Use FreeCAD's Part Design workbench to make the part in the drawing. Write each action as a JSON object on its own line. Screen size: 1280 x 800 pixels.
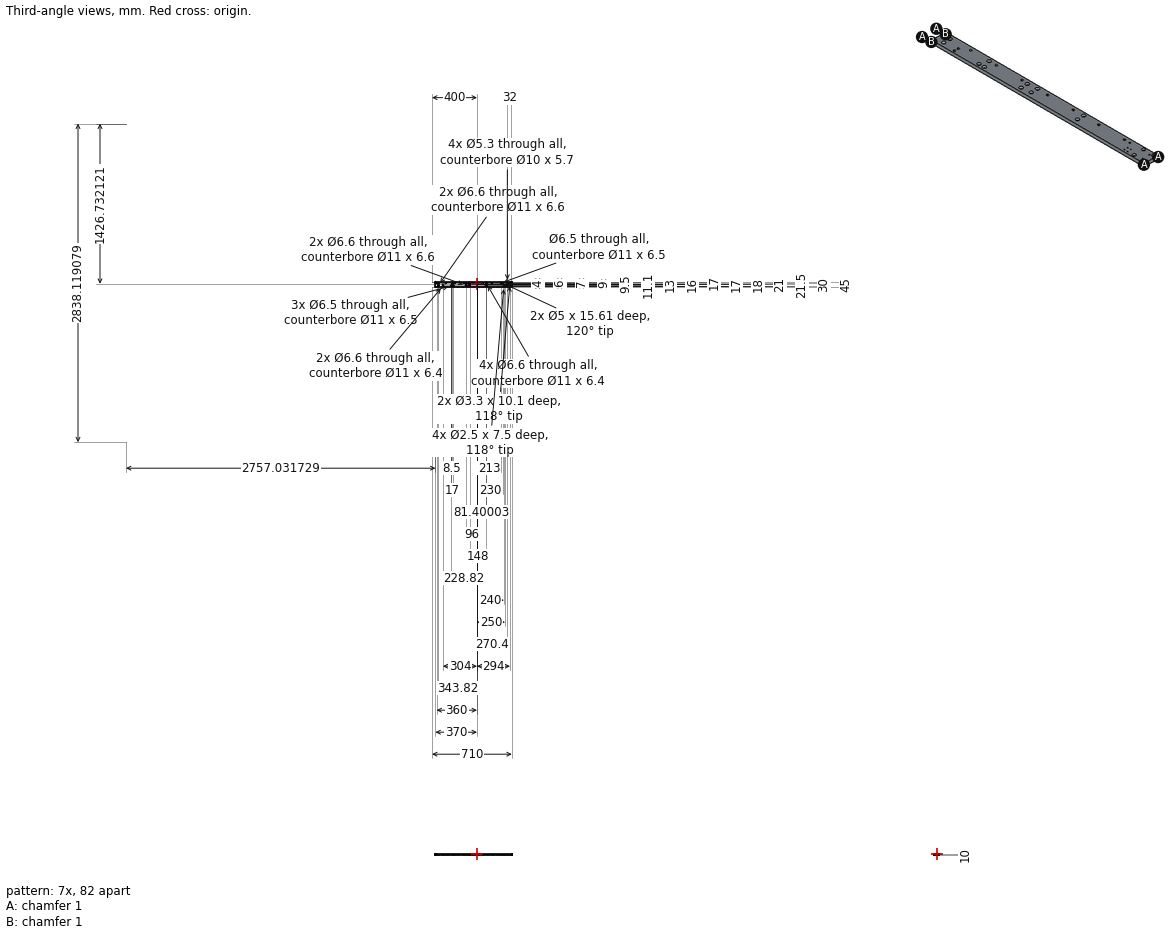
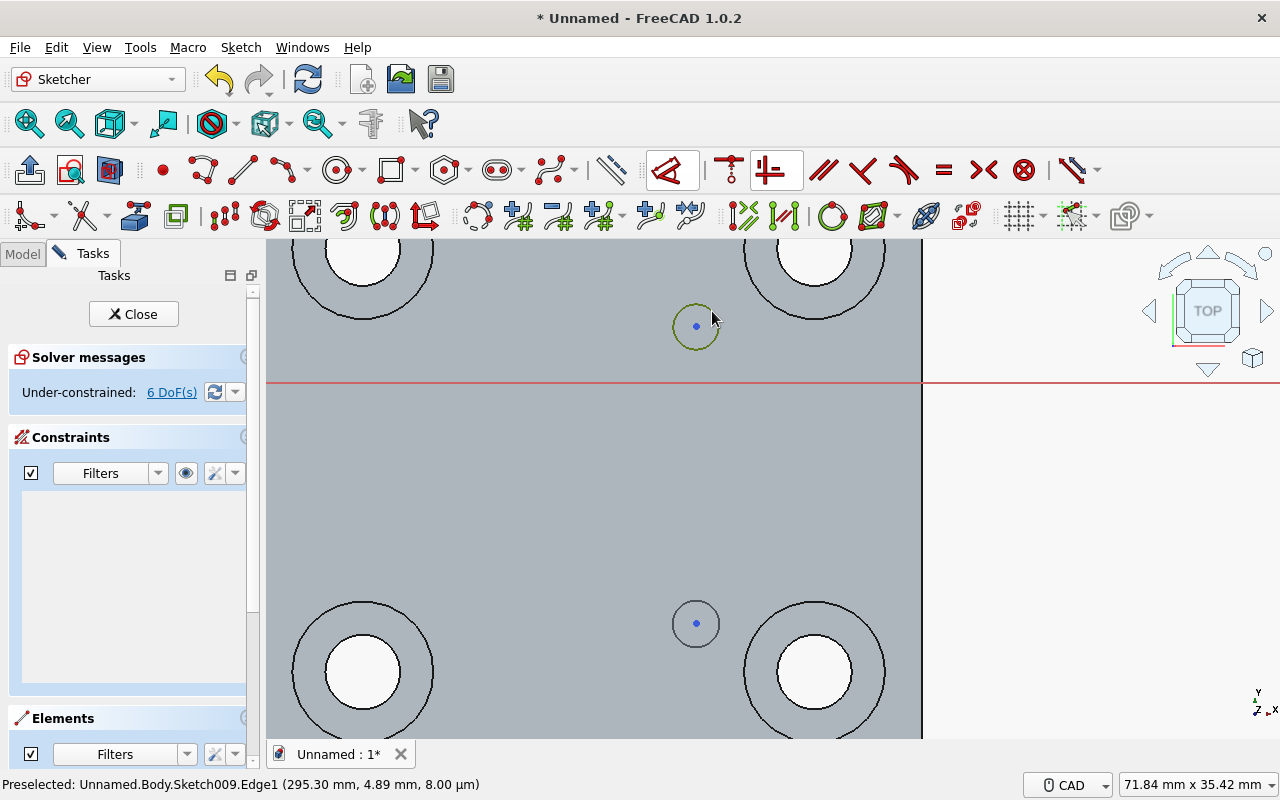
{"action": "left_click", "coordinate": [712, 607]}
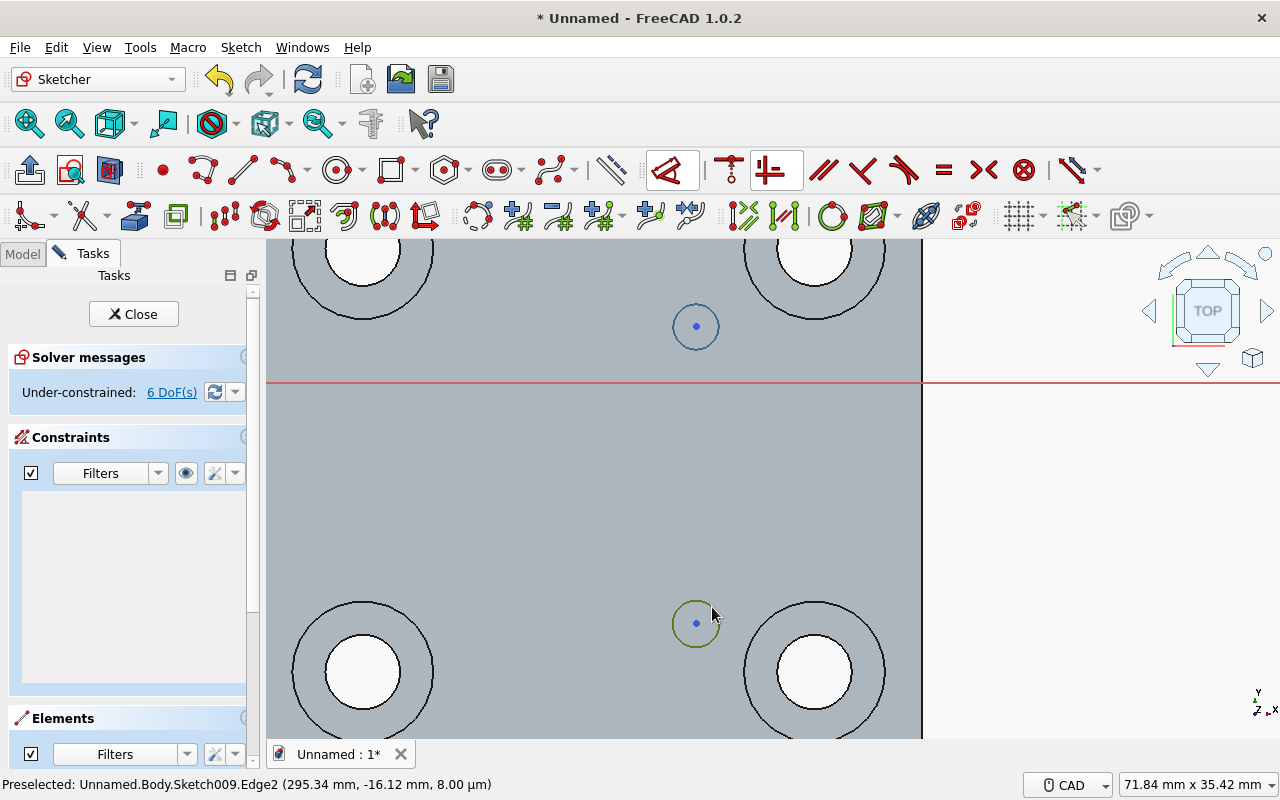
{"action": "left_click", "coordinate": [944, 170]}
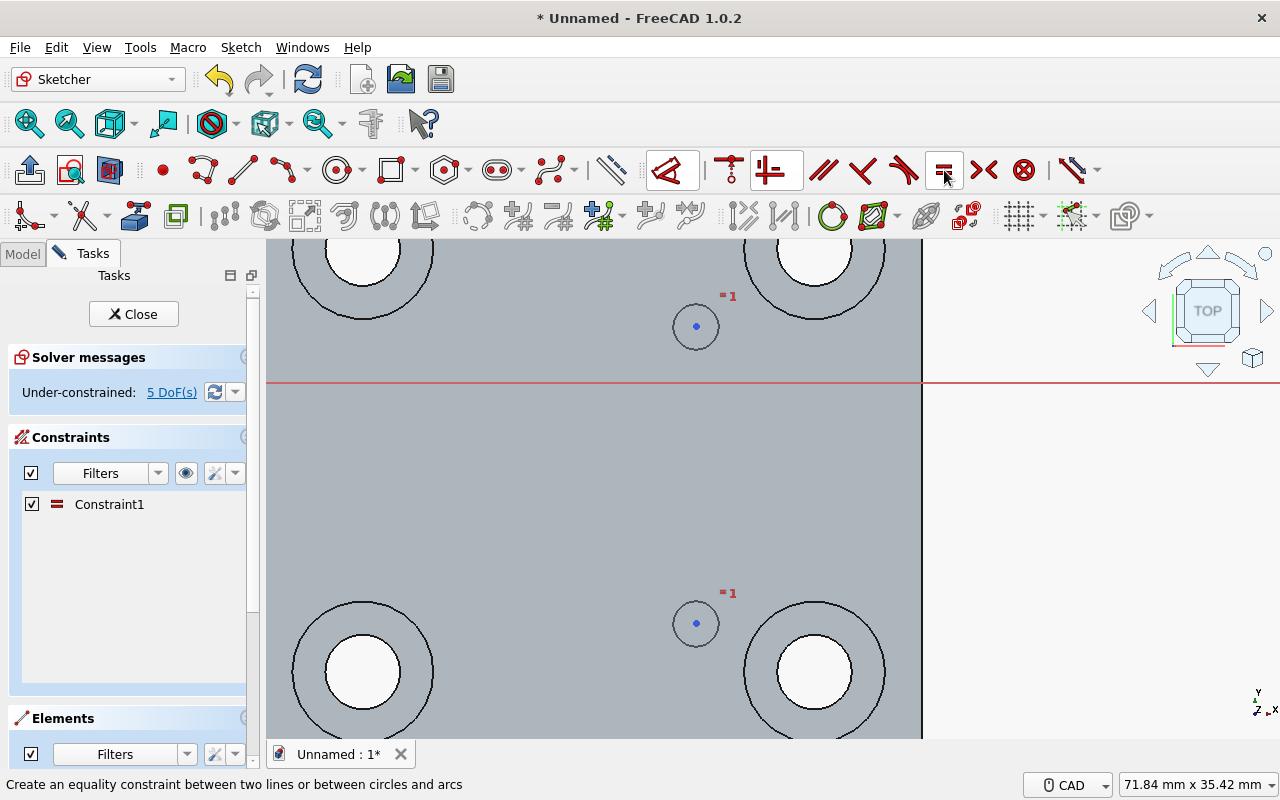
{"action": "left_click", "coordinate": [696, 327]}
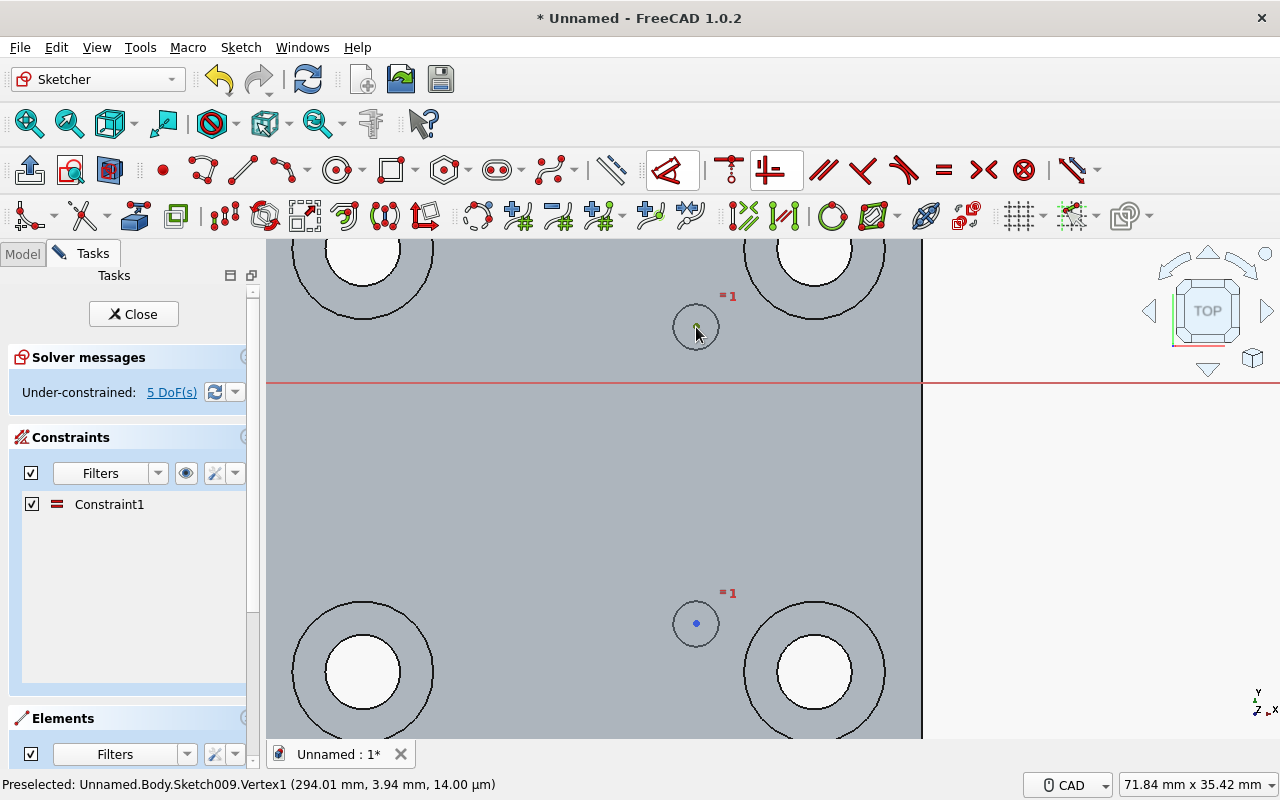
{"action": "left_click", "coordinate": [696, 624]}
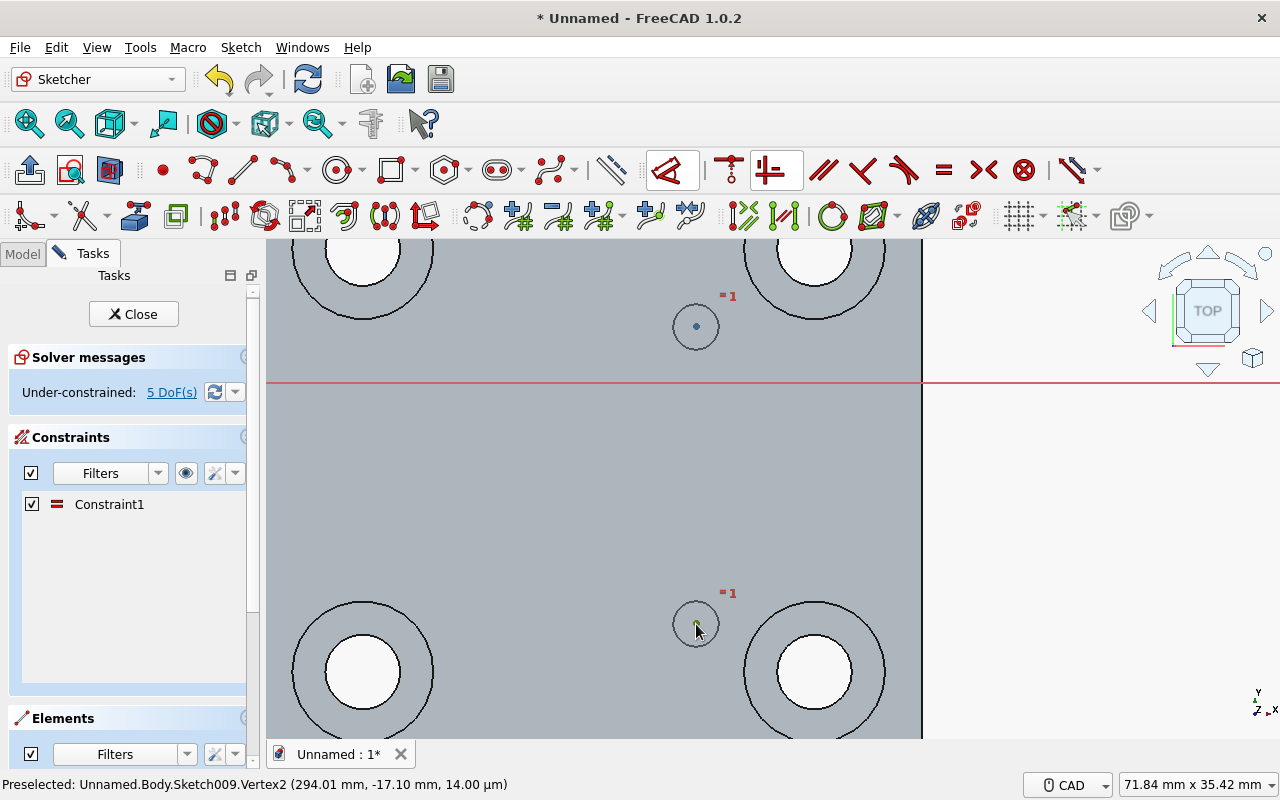
{"action": "left_click", "coordinate": [798, 170]}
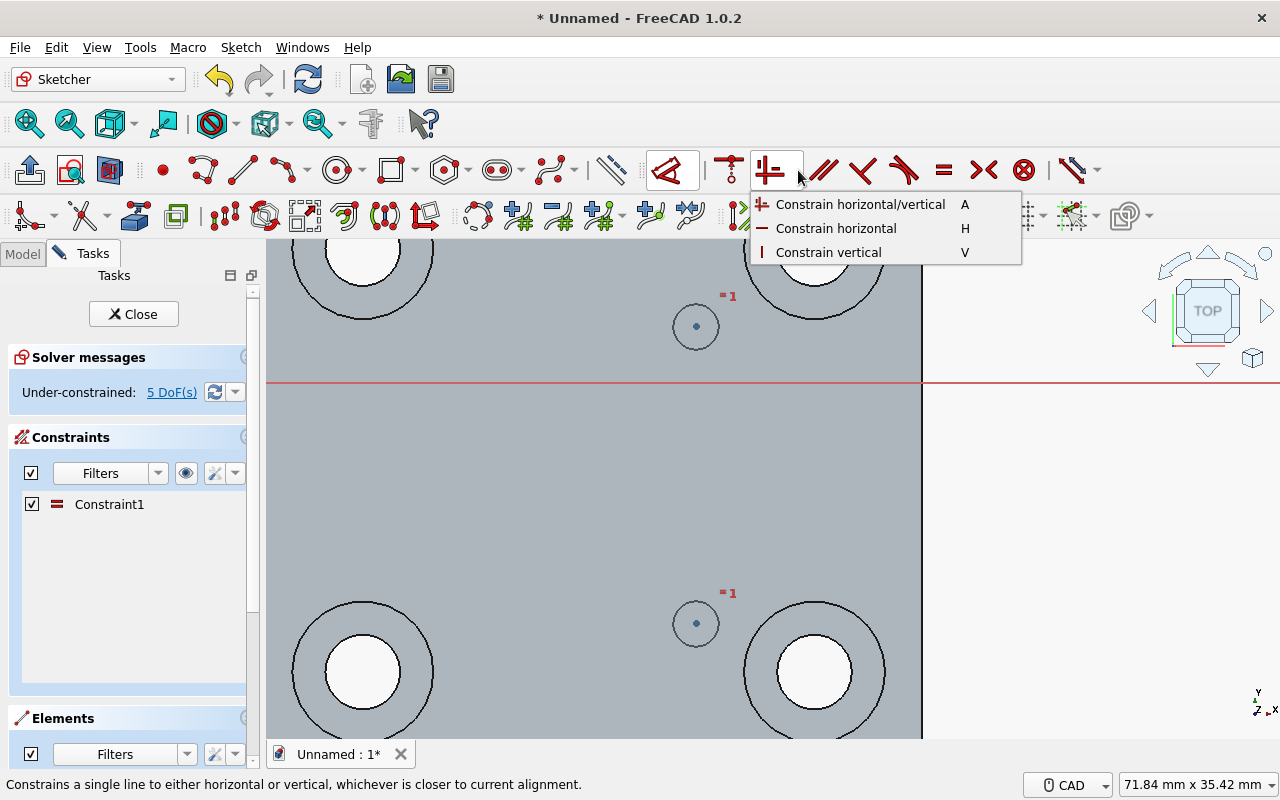
{"action": "left_click", "coordinate": [886, 252]}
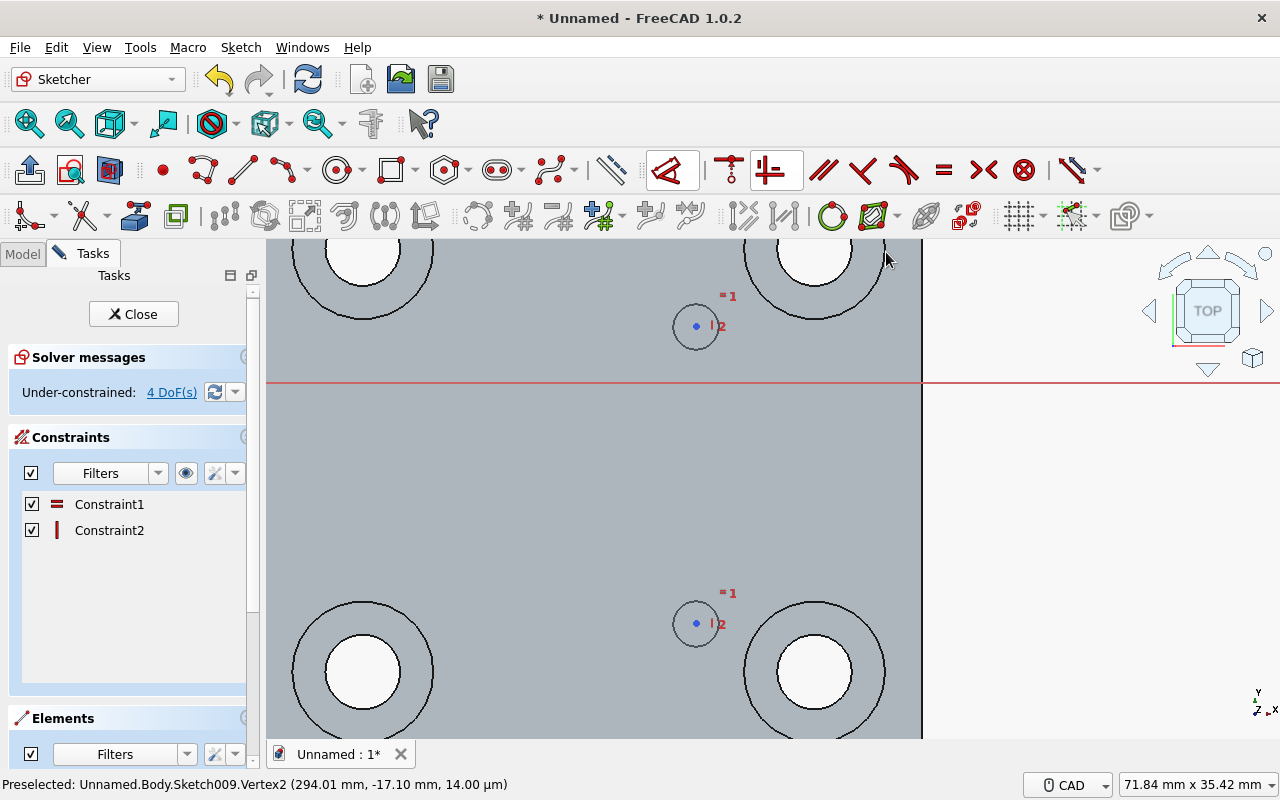
{"action": "left_click", "coordinate": [712, 311]}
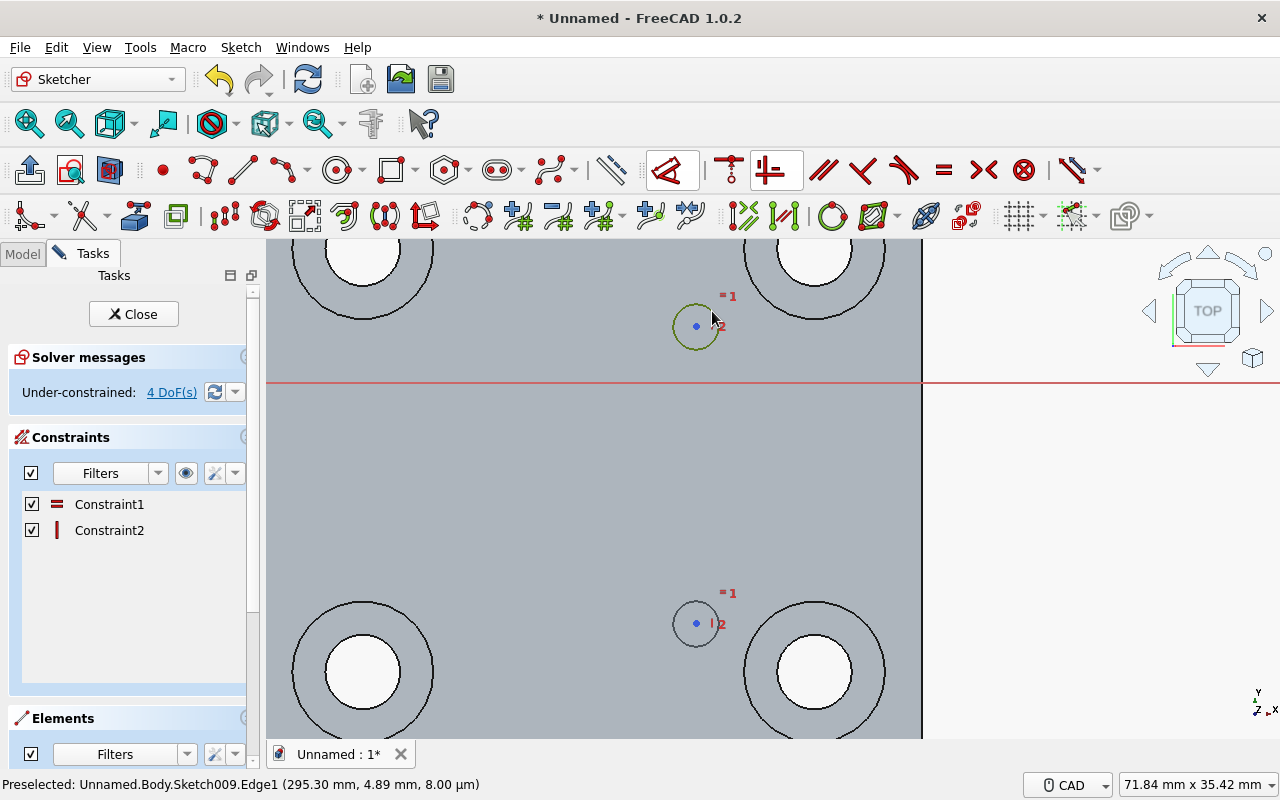
{"action": "left_click", "coordinate": [694, 170]}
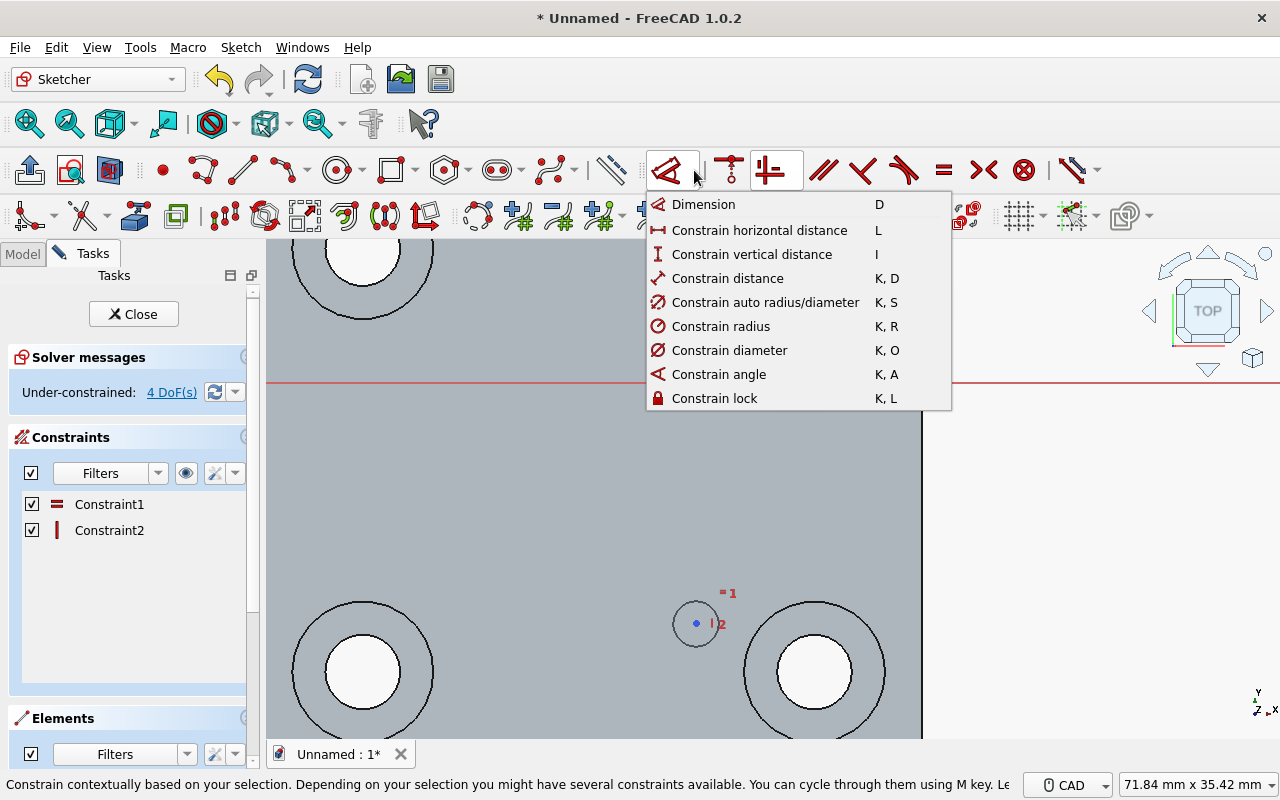
{"action": "left_click", "coordinate": [799, 350]}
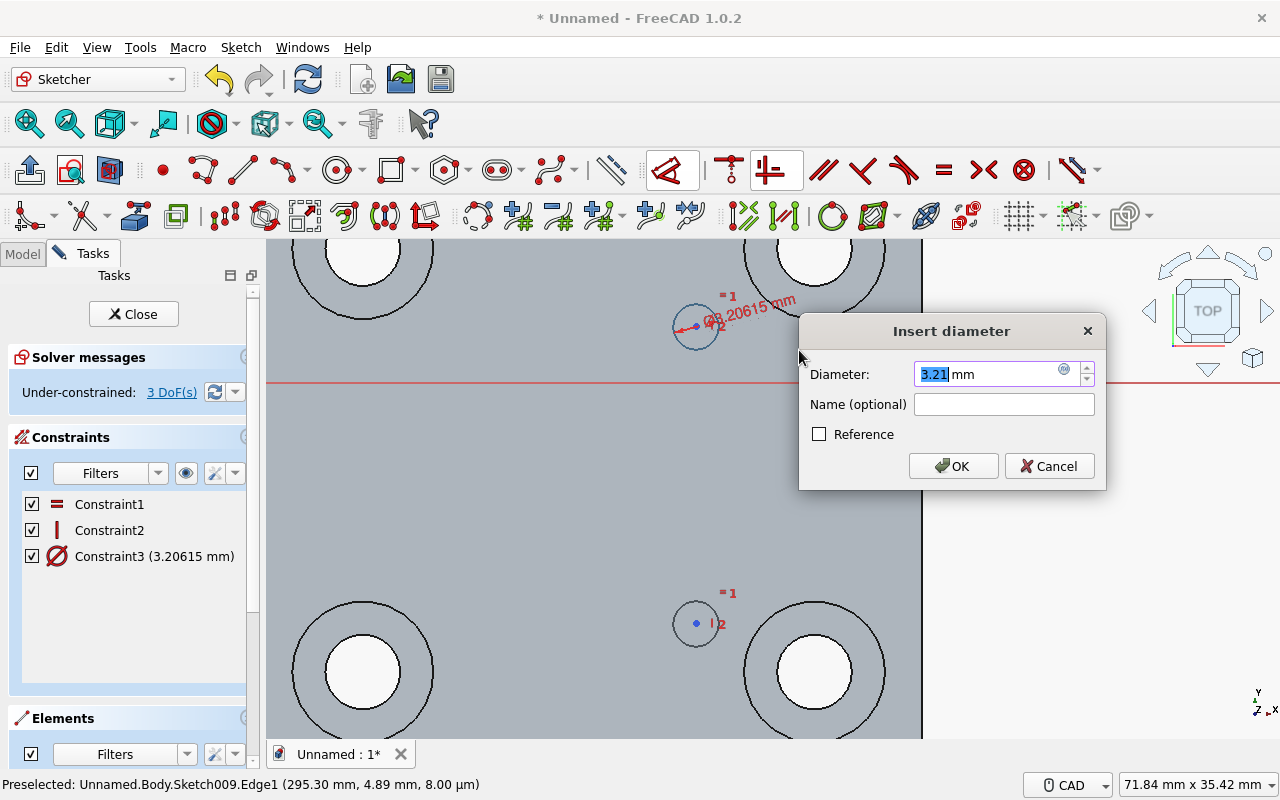
{"action": "type", "text": "3.3"}
{"action": "key", "text": "Return"}